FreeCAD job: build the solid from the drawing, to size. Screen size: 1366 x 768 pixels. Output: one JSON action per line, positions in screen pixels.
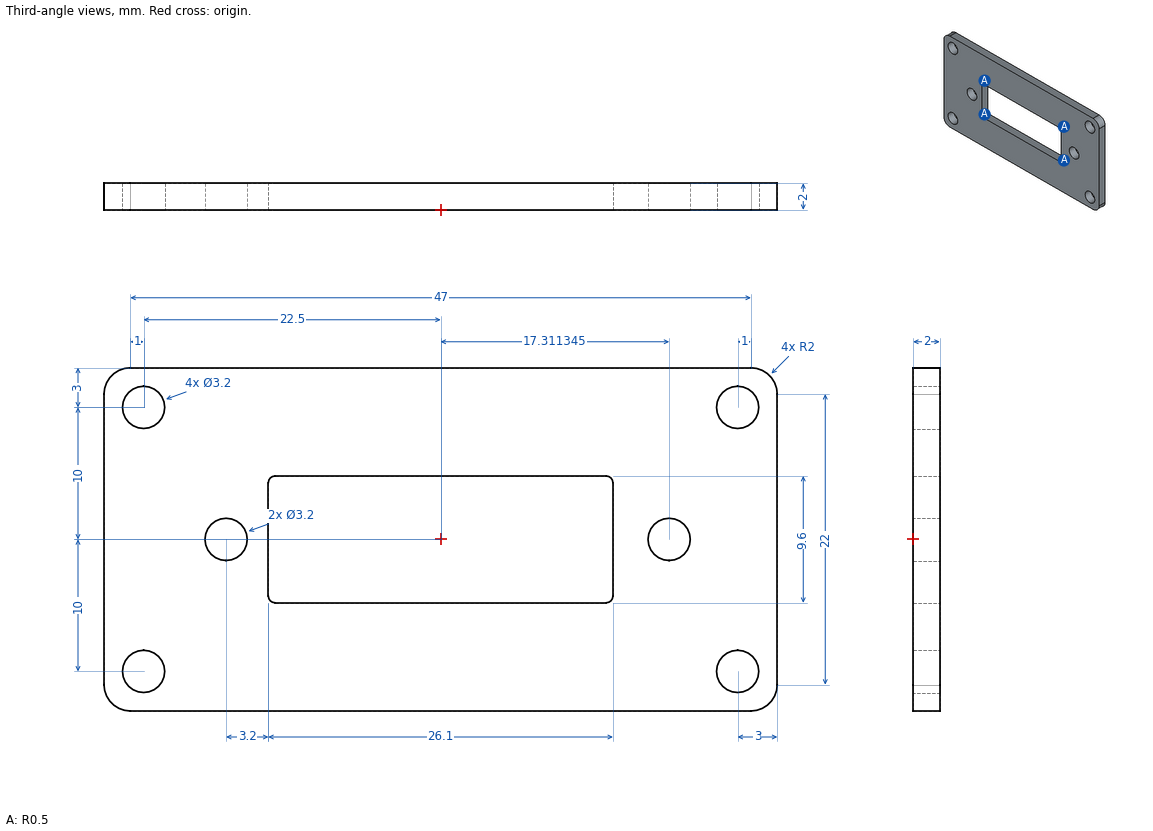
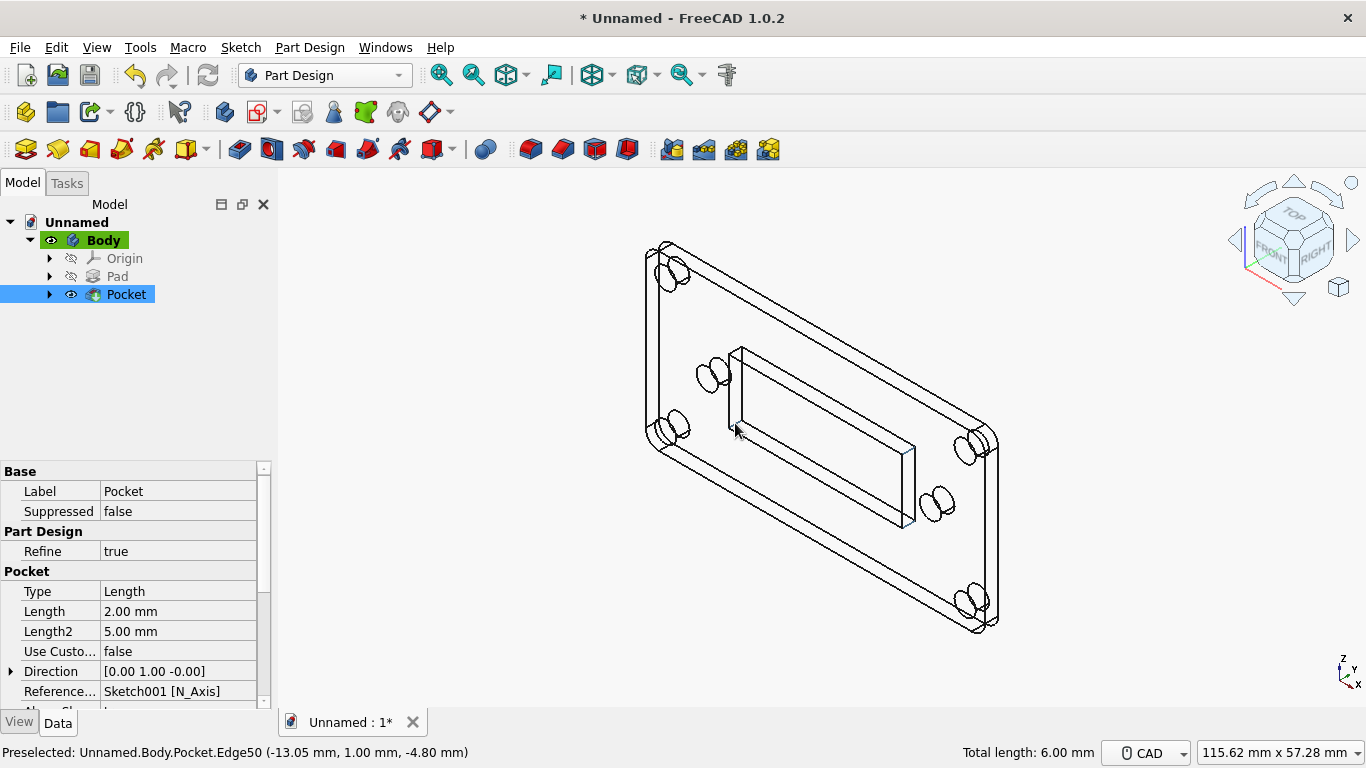
{"action": "left_click", "coordinate": [735, 349], "text": "ctrl"}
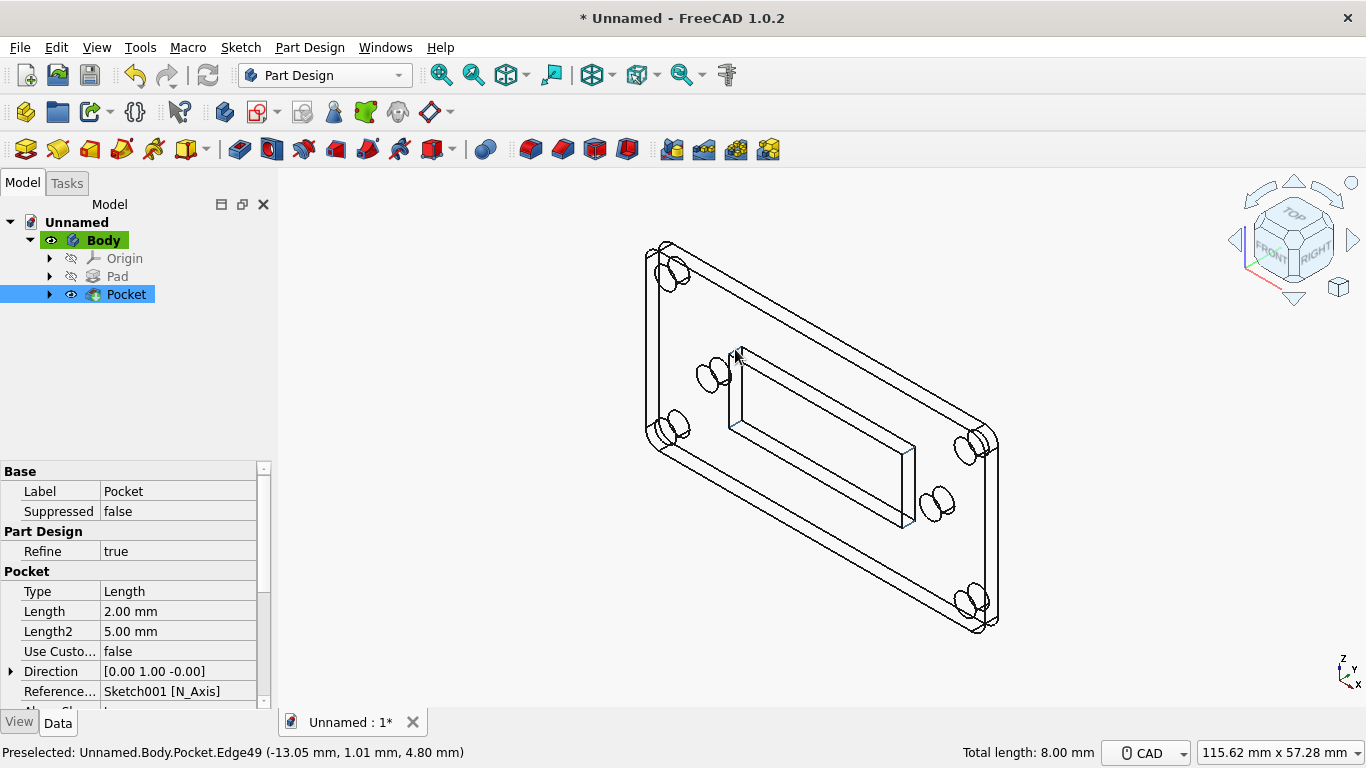
{"action": "key", "text": "v 1"}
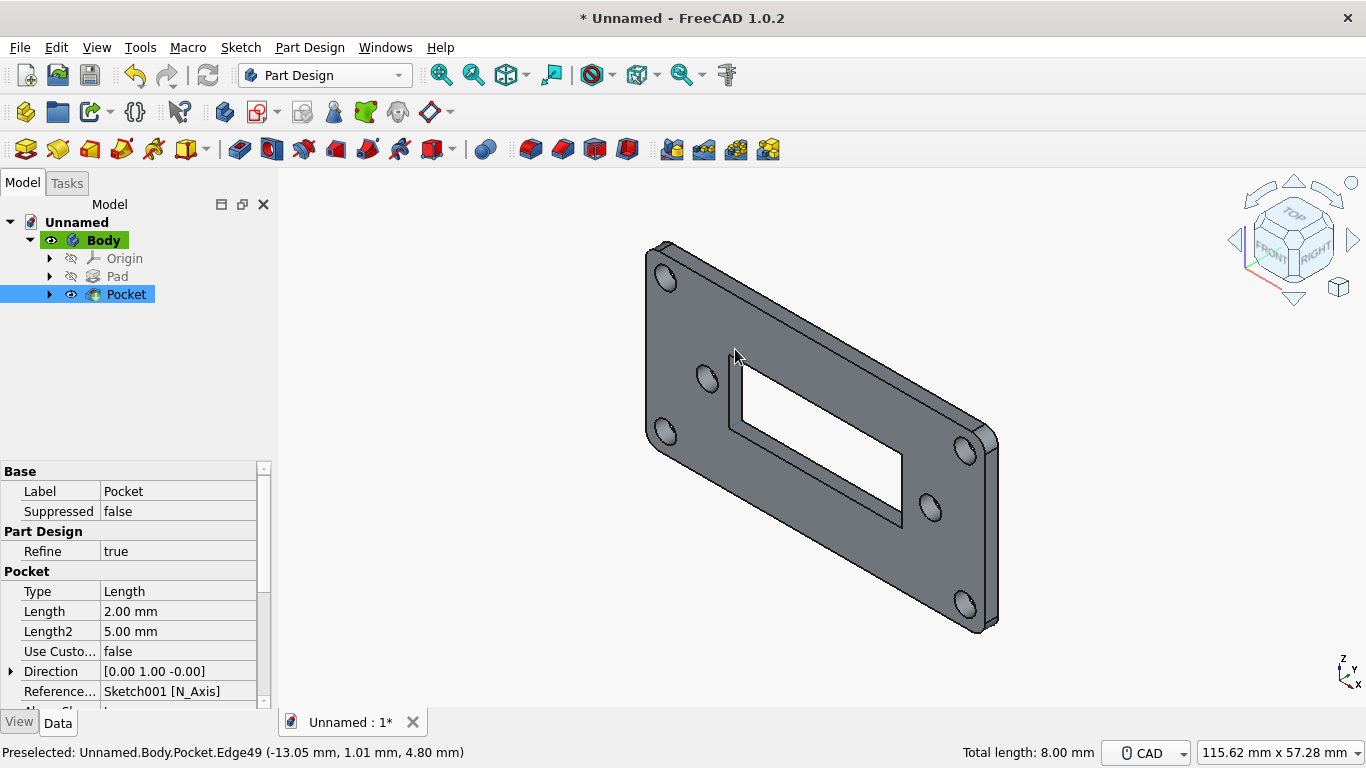
{"action": "left_click", "coordinate": [532, 150]}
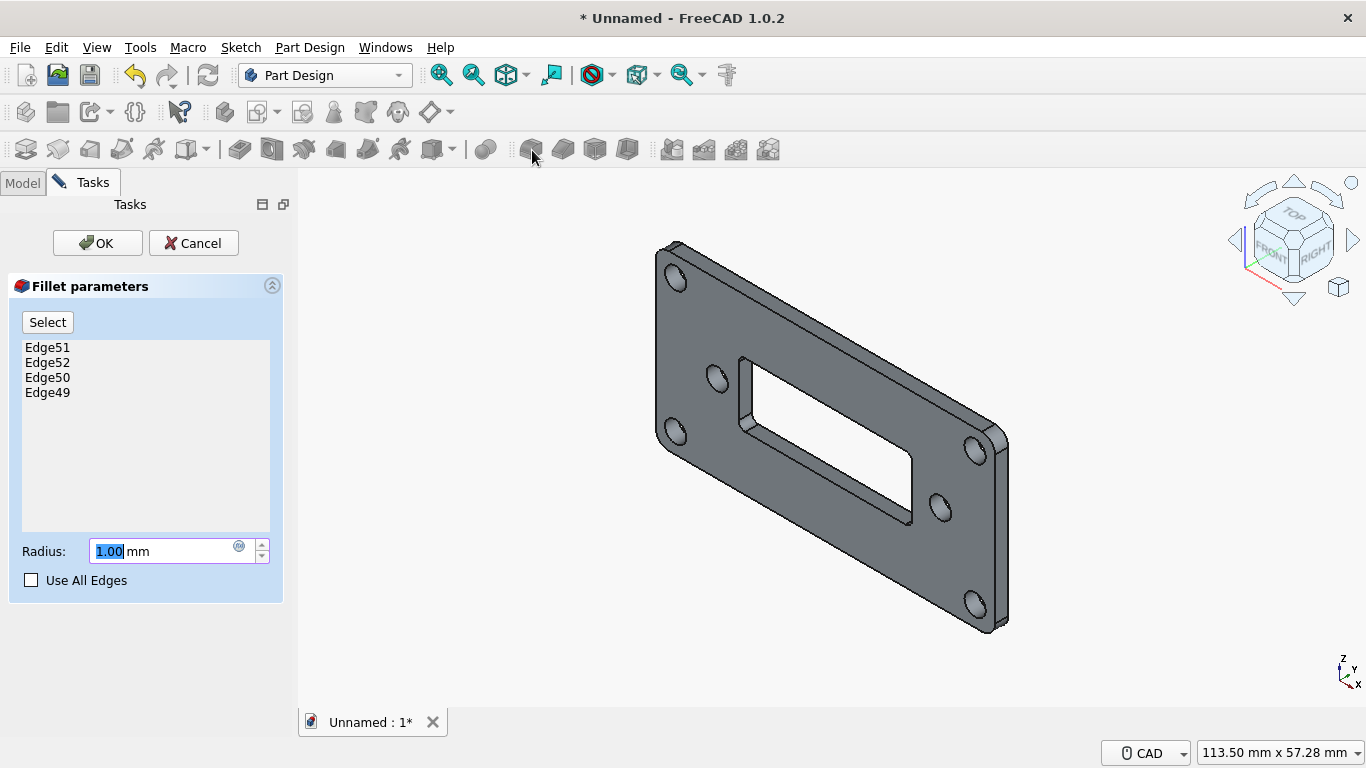
{"action": "type", "text": "0.5"}
{"action": "key", "text": "Tab"}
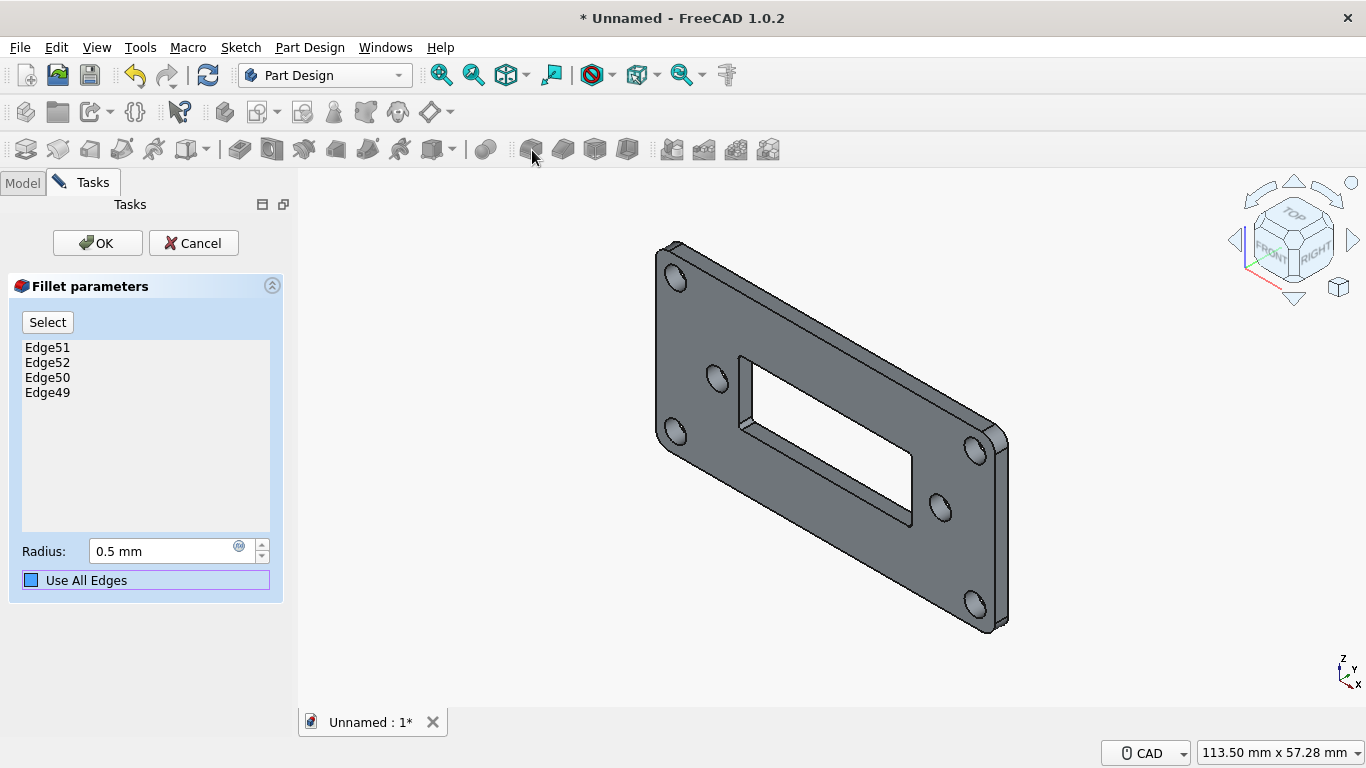
{"action": "left_click", "coordinate": [98, 243]}